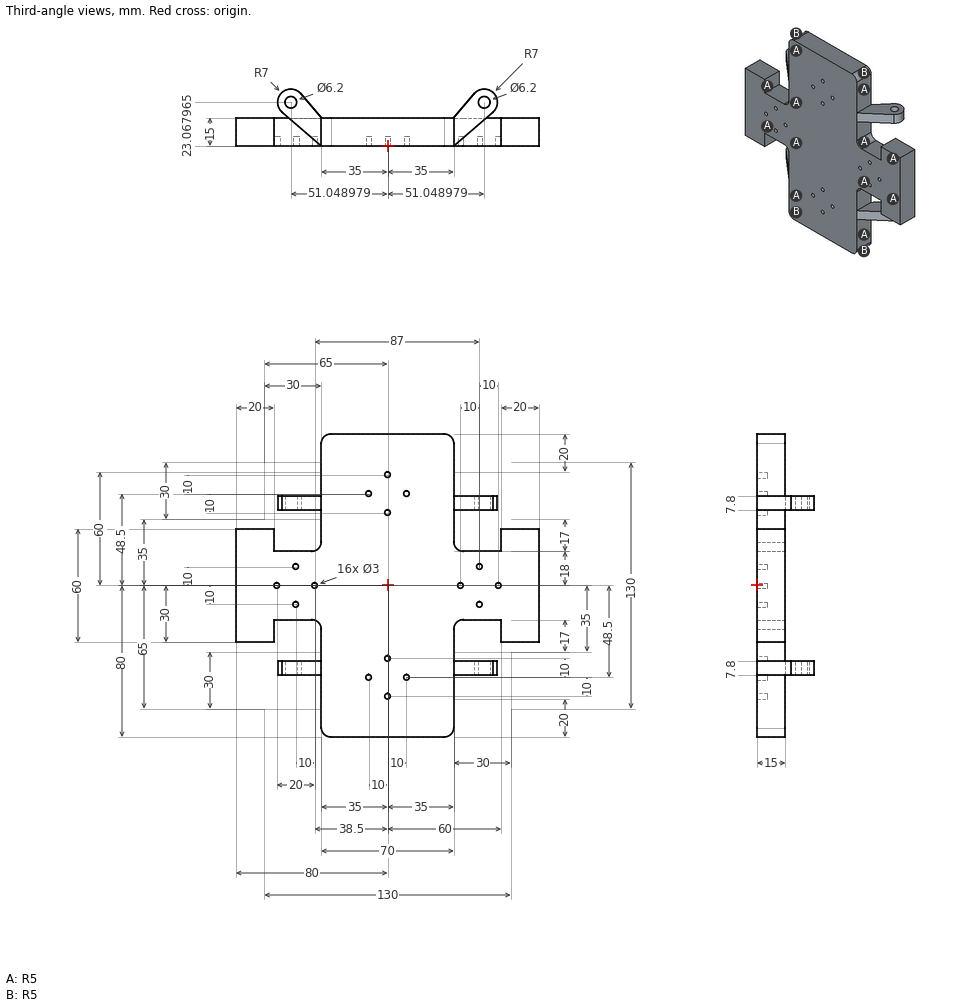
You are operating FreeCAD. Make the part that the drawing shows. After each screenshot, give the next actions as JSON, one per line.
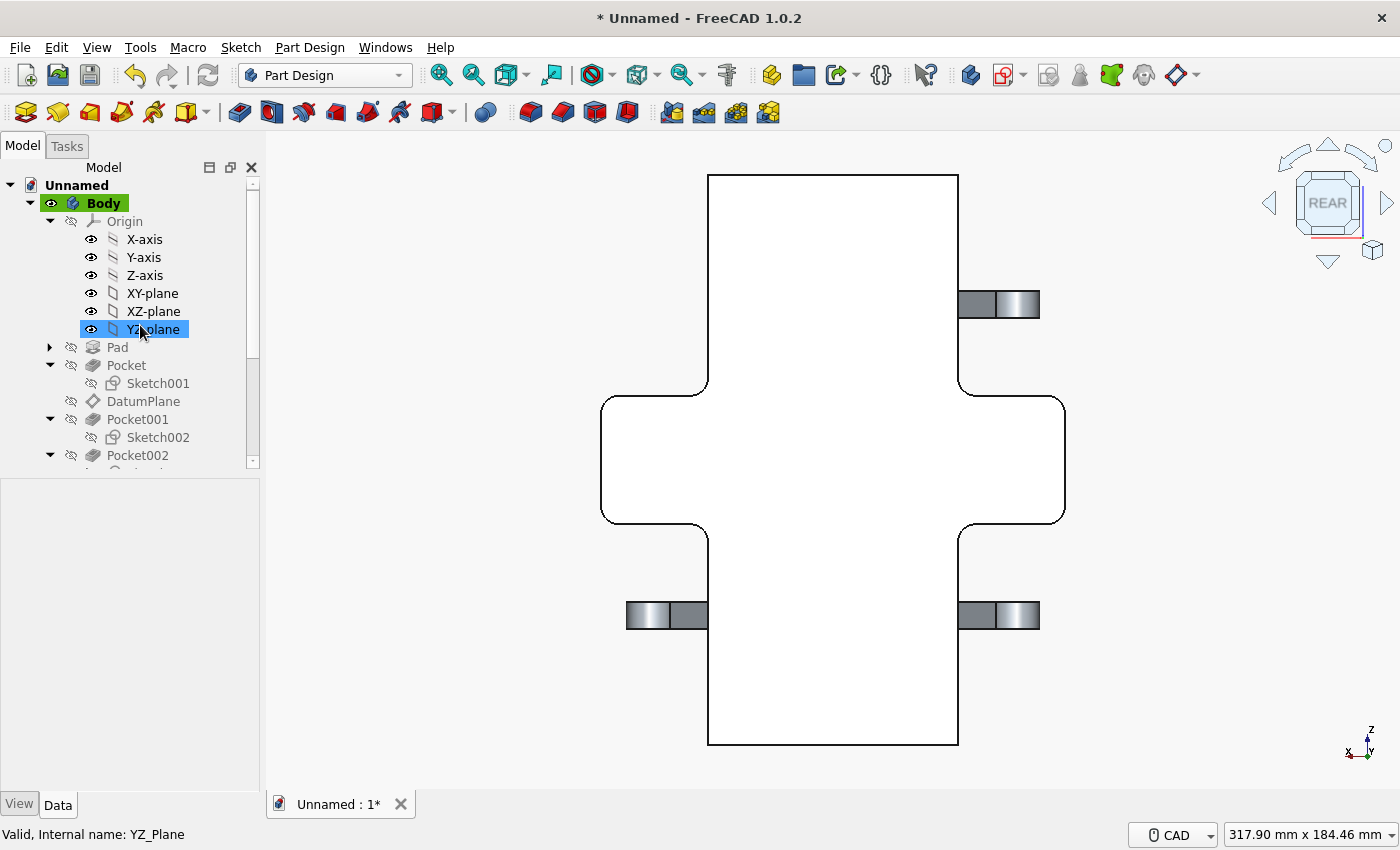
{"action": "left_click", "coordinate": [136, 293]}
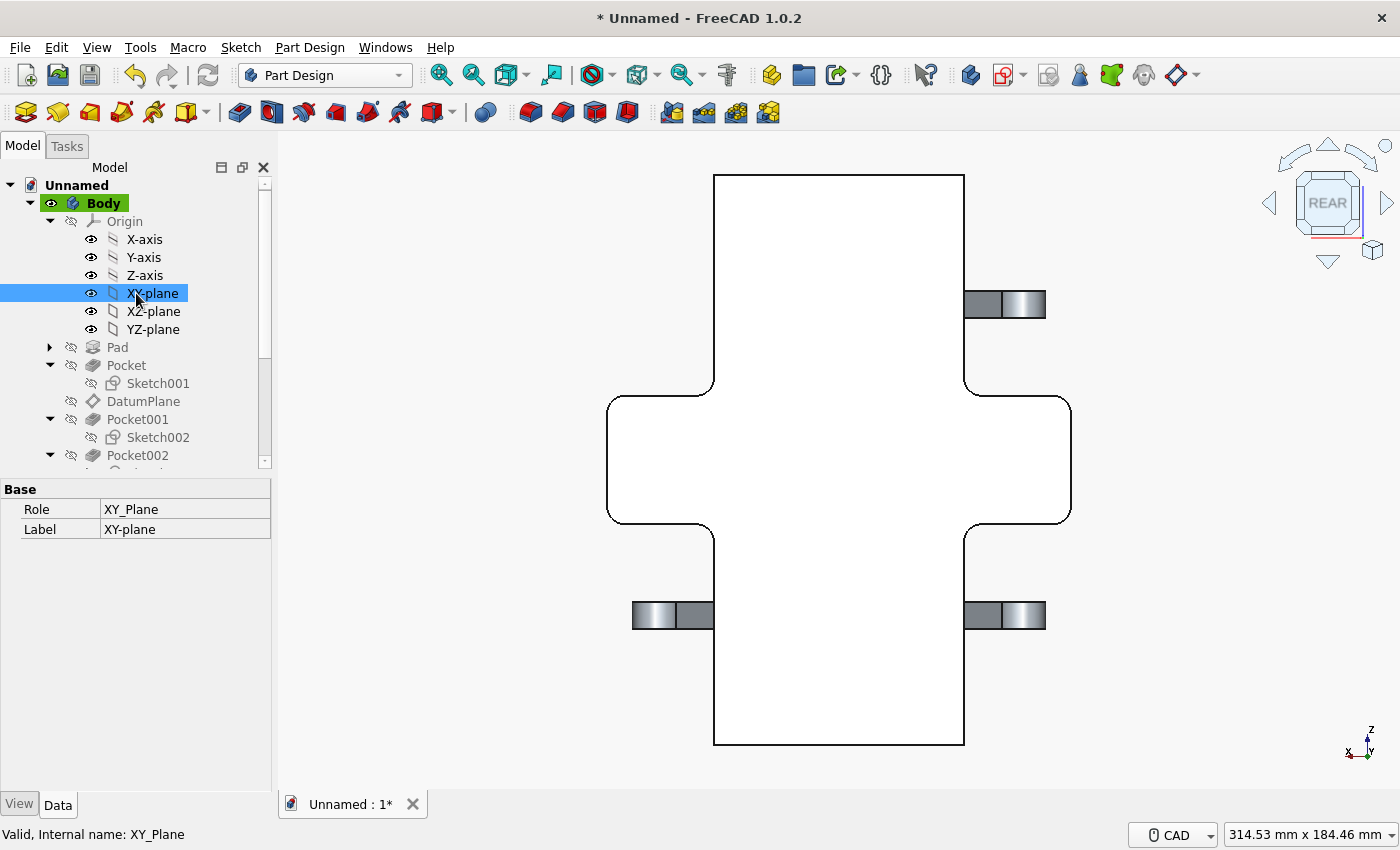
{"action": "left_click", "coordinate": [1176, 76]}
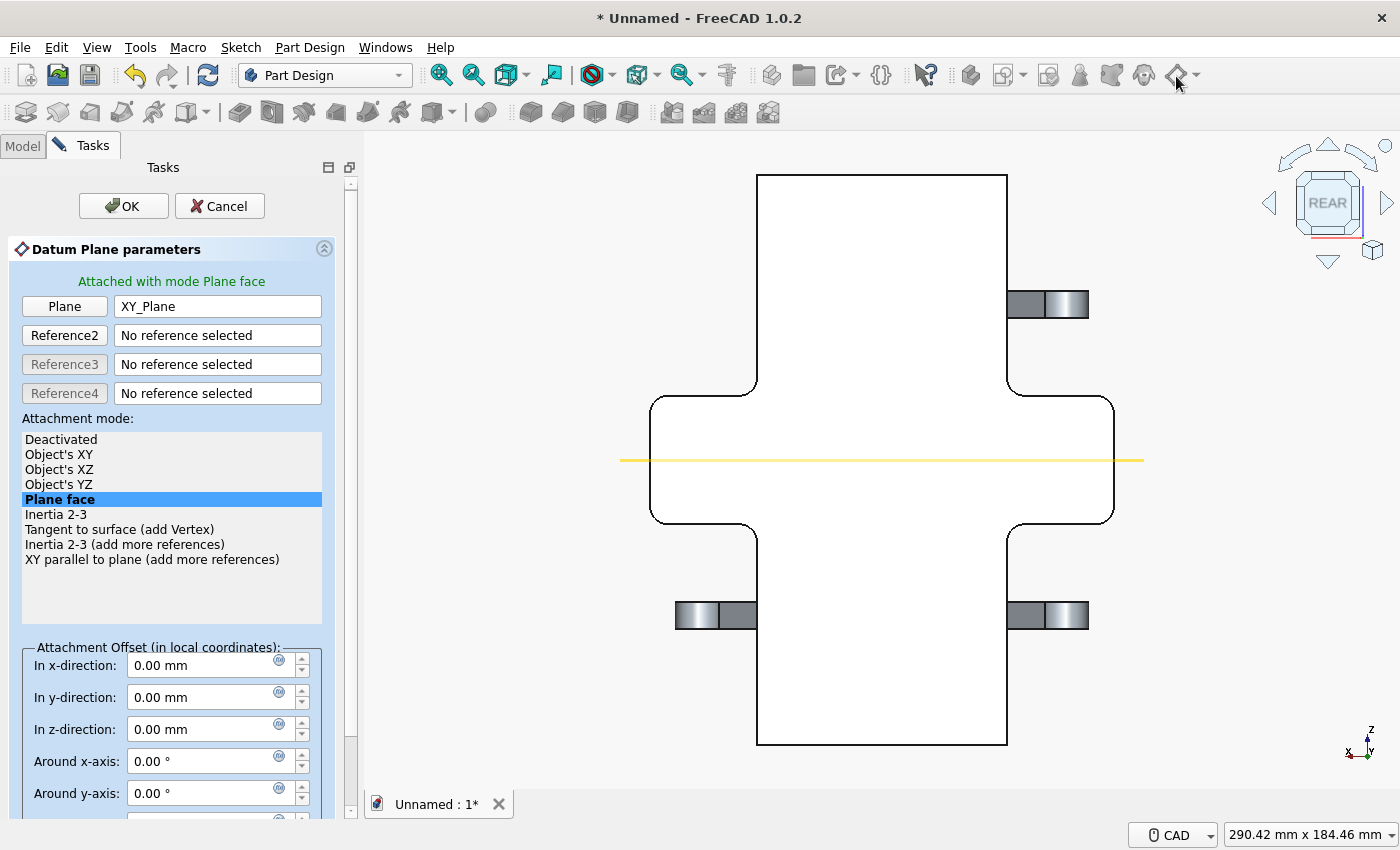
{"action": "triple_click", "coordinate": [210, 729]}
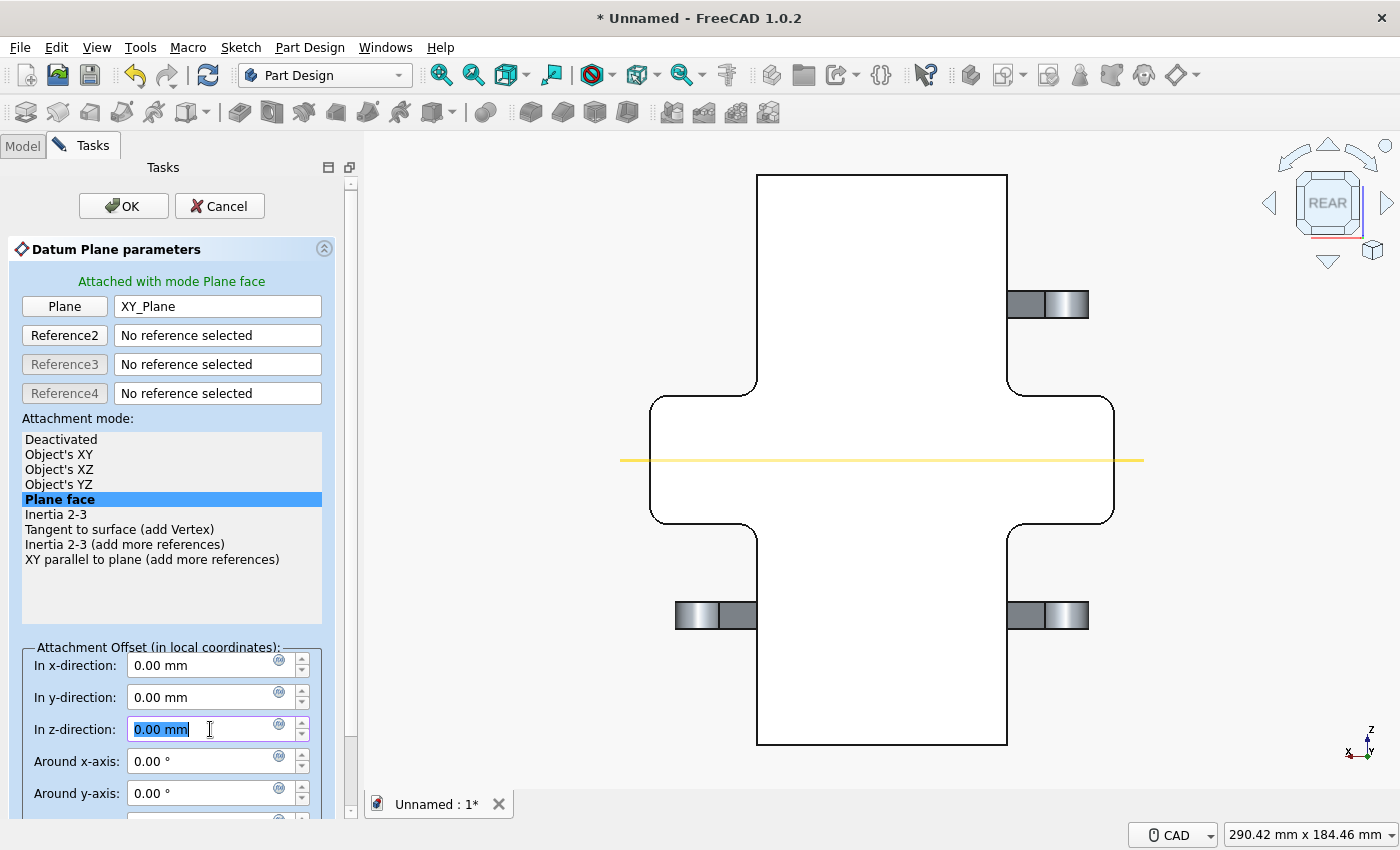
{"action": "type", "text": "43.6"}
{"action": "key", "text": "Tab"}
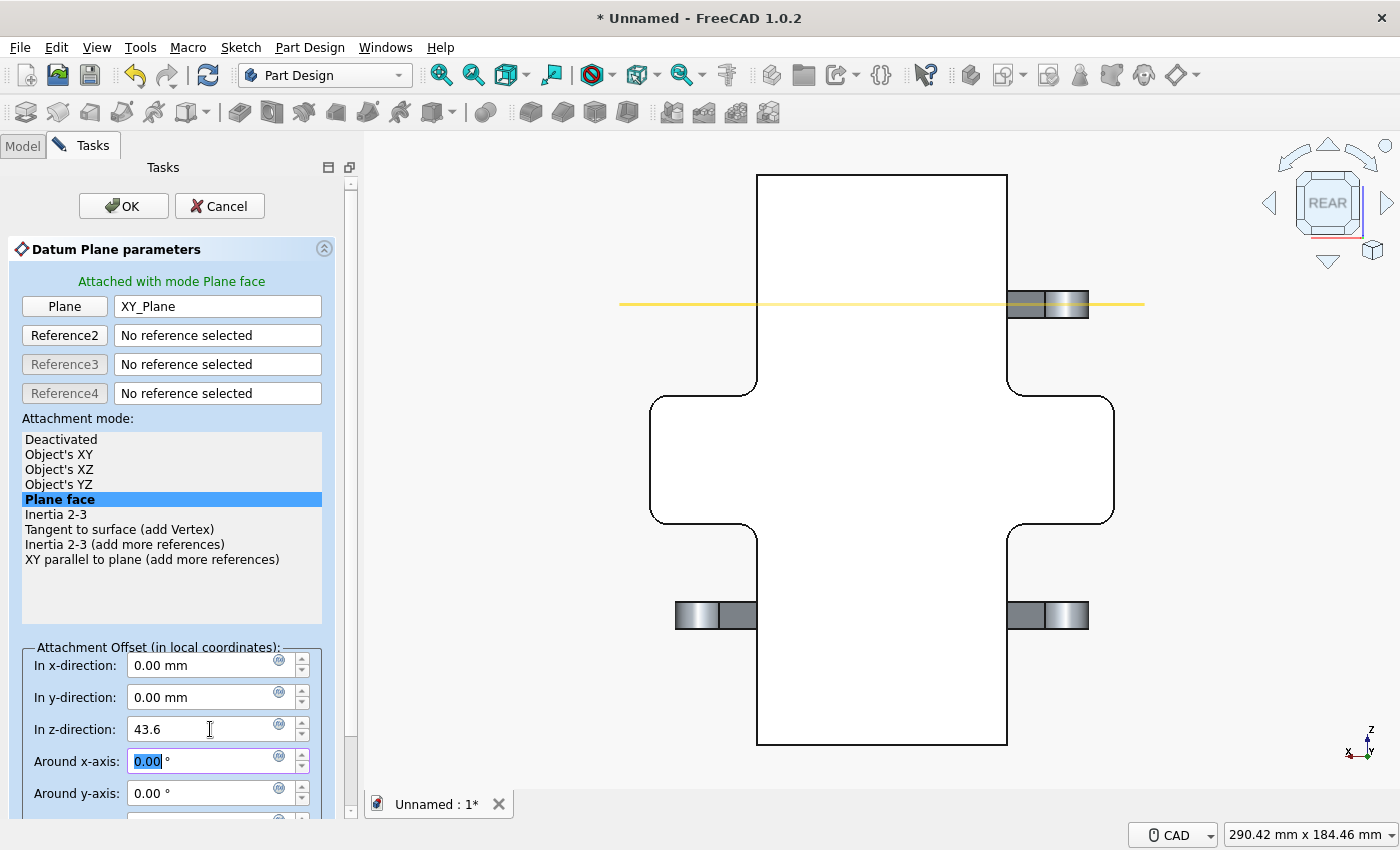
{"action": "left_click", "coordinate": [124, 206]}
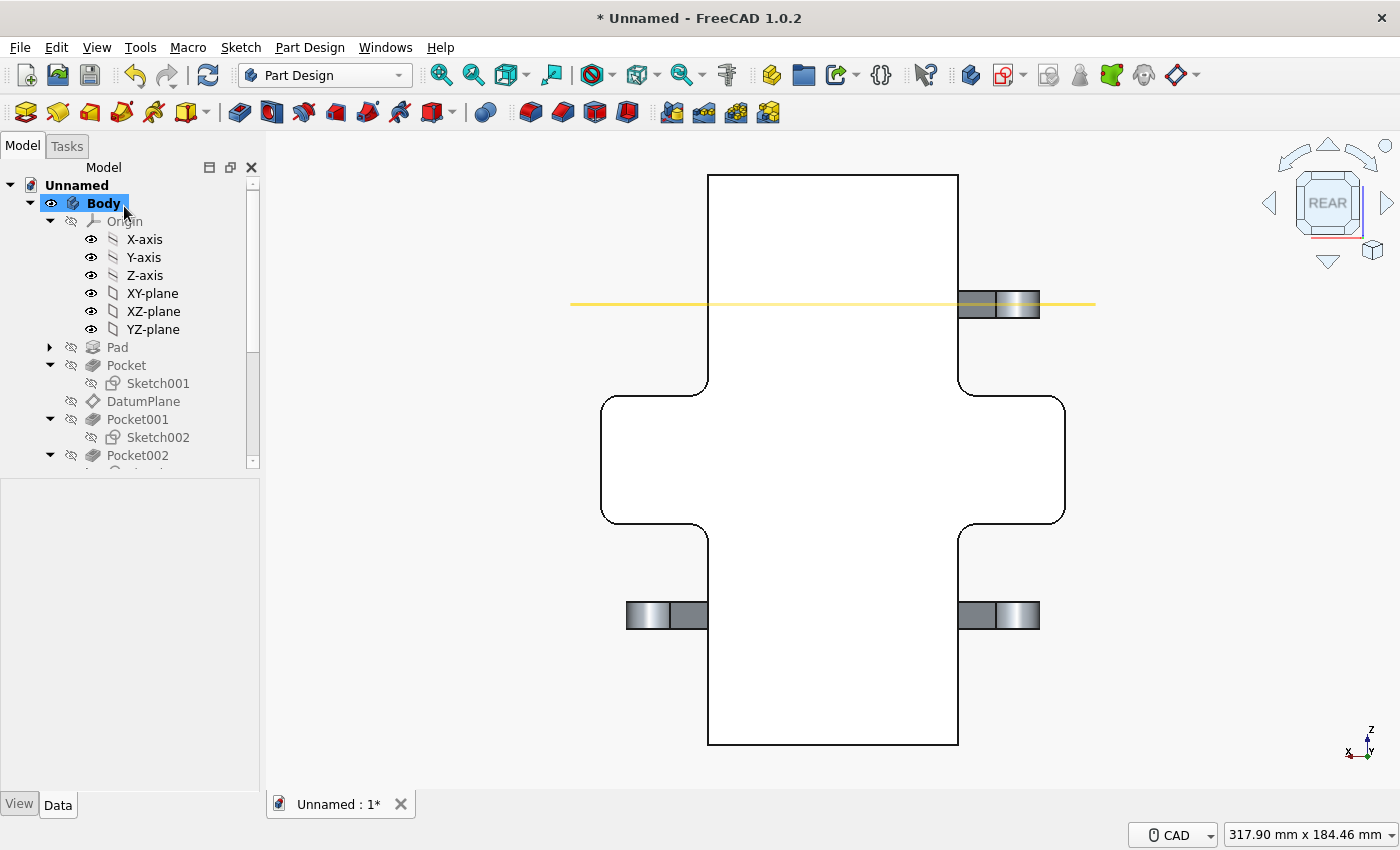
{"action": "scroll", "coordinate": [100, 325], "scroll_direction": "down", "scroll_amount": 3}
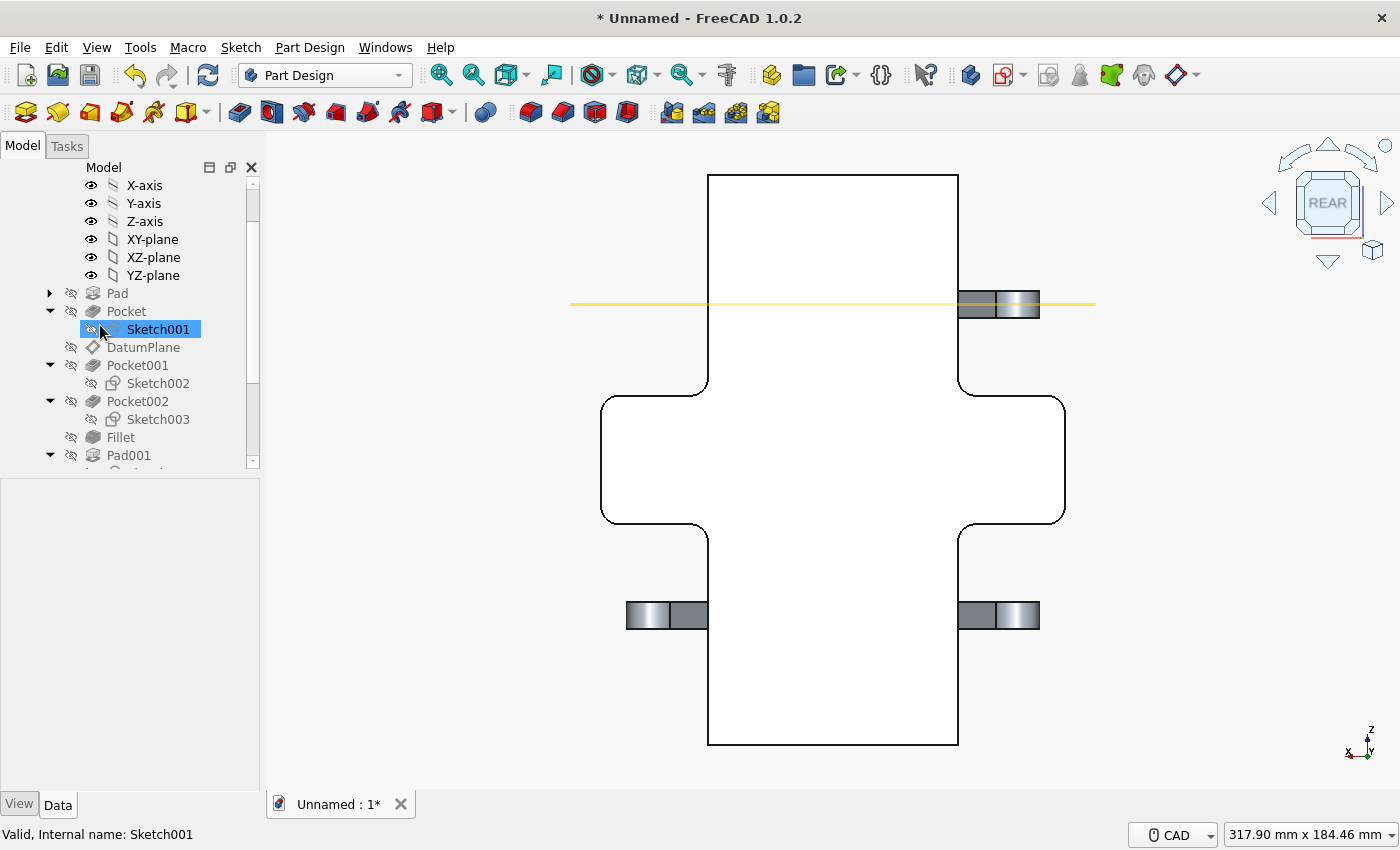
{"action": "scroll", "coordinate": [140, 325], "scroll_direction": "up", "scroll_amount": 15}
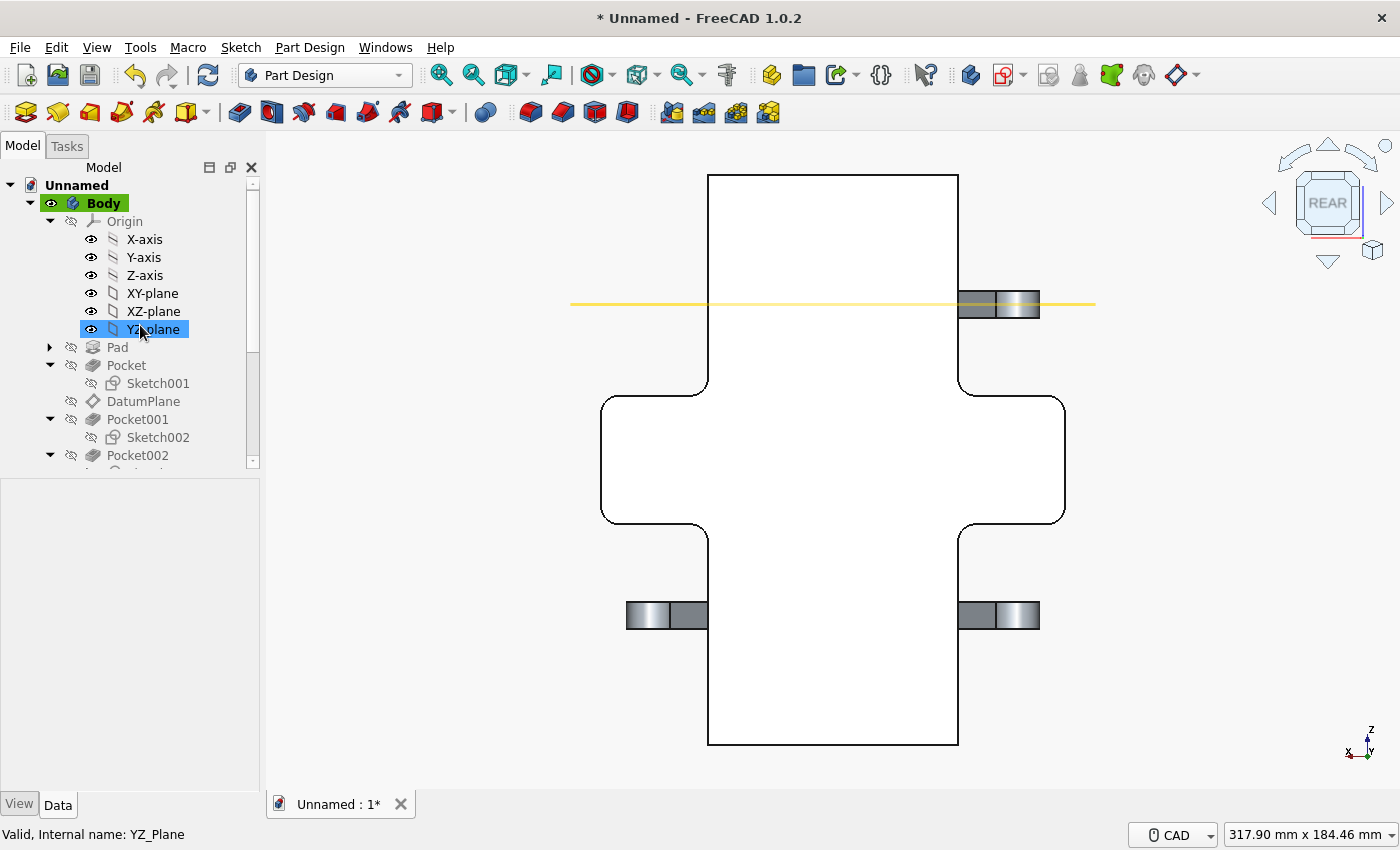
{"action": "scroll", "coordinate": [100, 325], "scroll_direction": "down", "scroll_amount": 6}